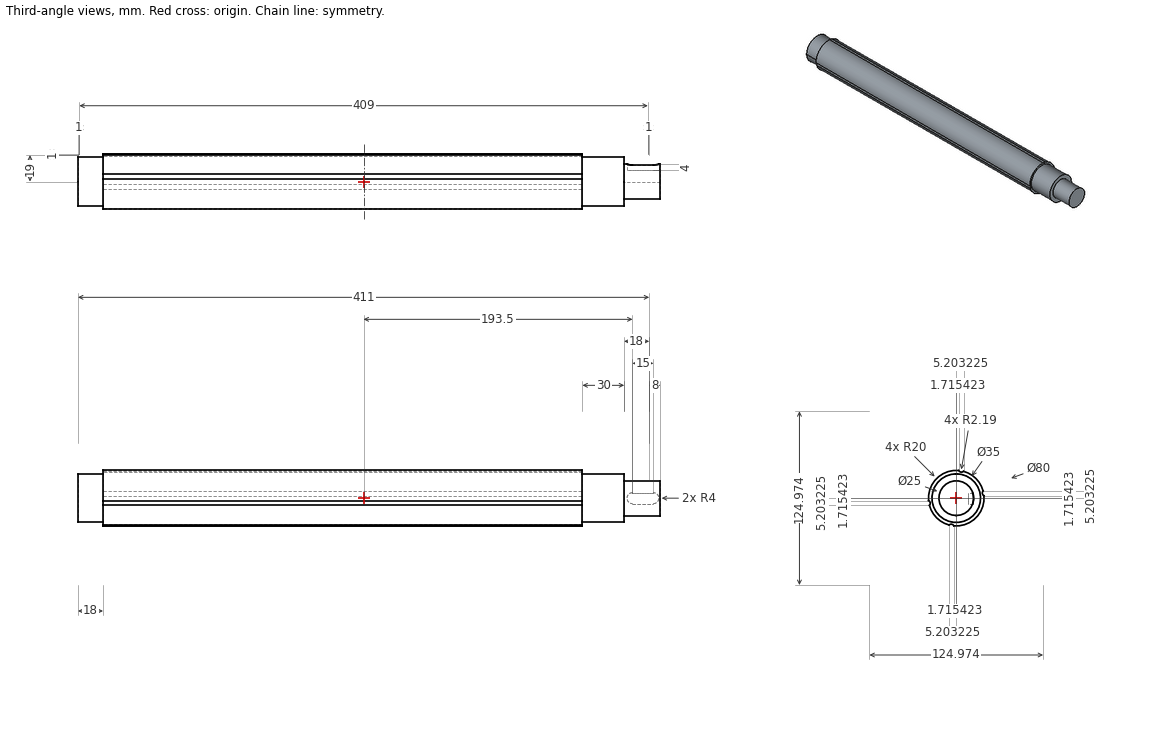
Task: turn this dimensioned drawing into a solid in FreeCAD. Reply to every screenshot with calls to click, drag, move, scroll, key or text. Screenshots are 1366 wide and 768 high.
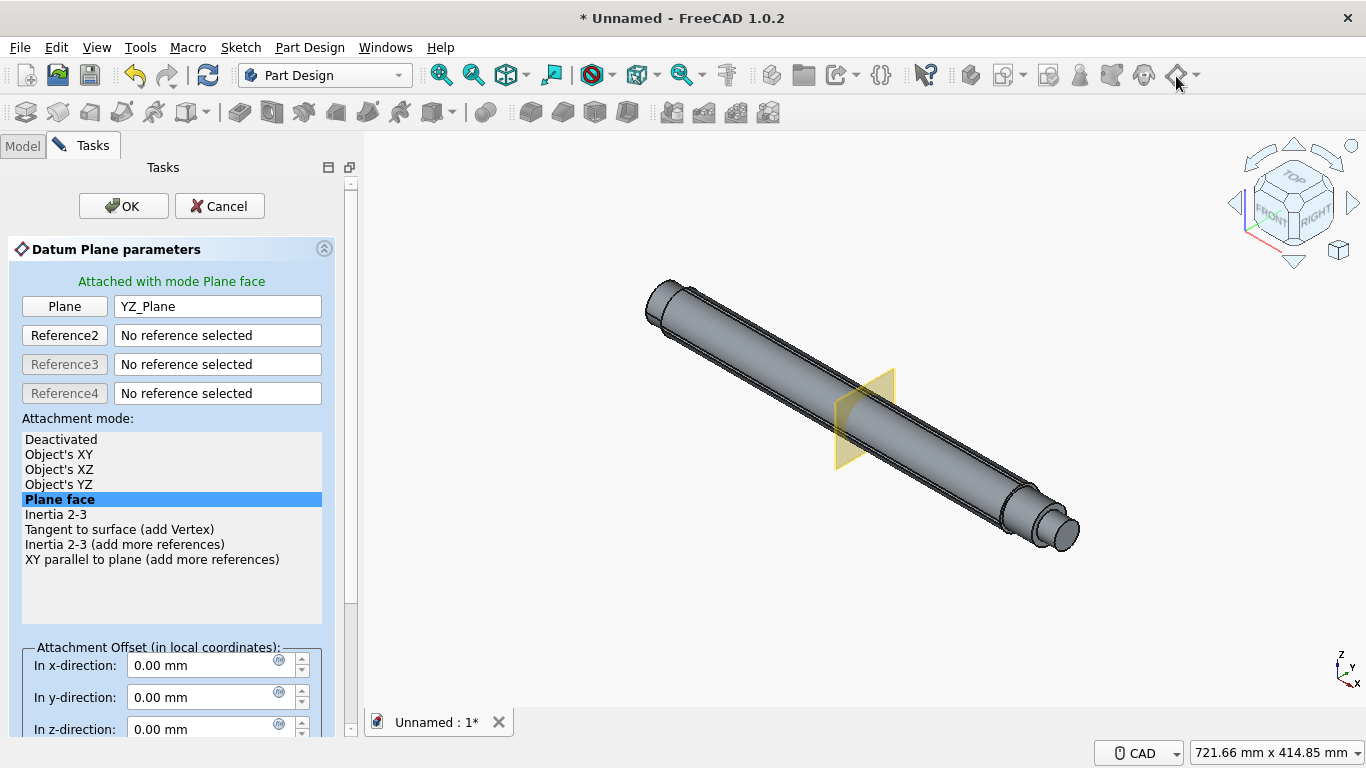
scroll(351, 456, down, 2)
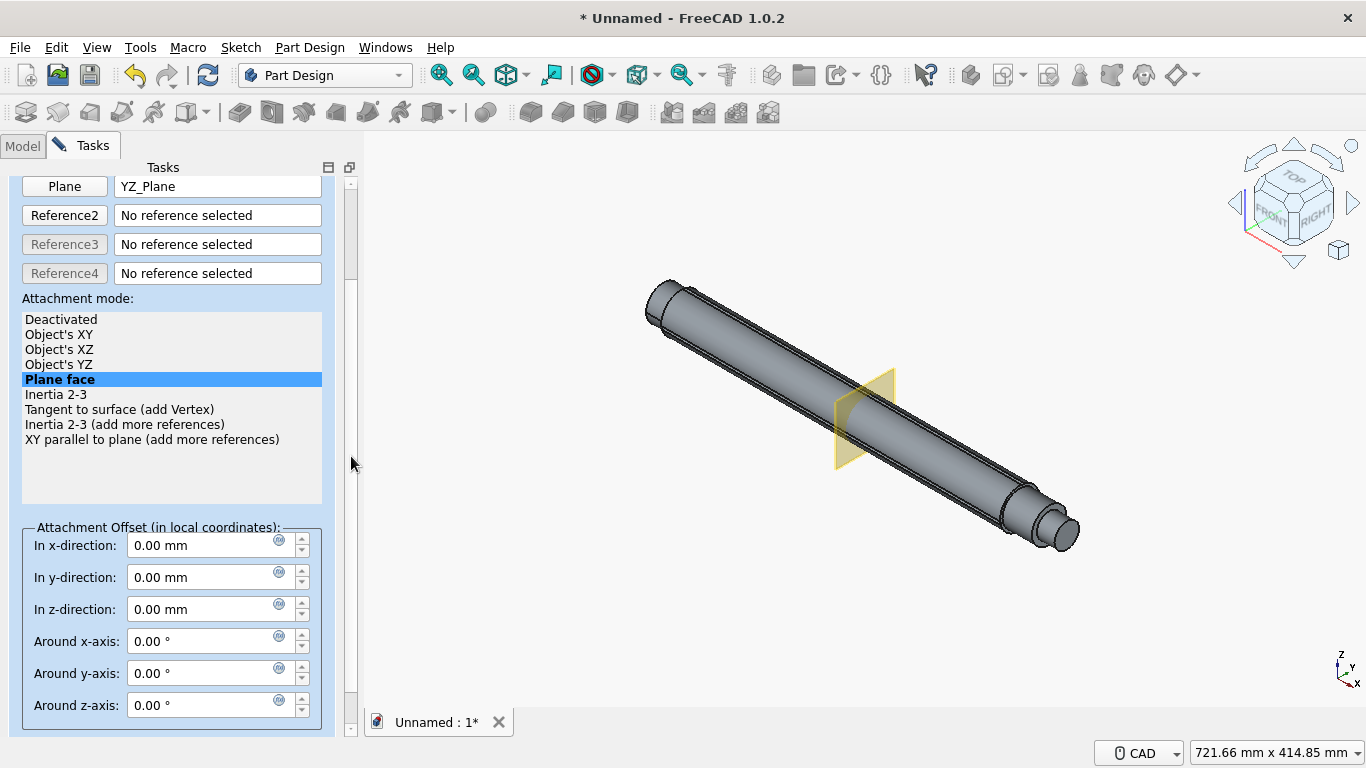
triple_click(210, 609)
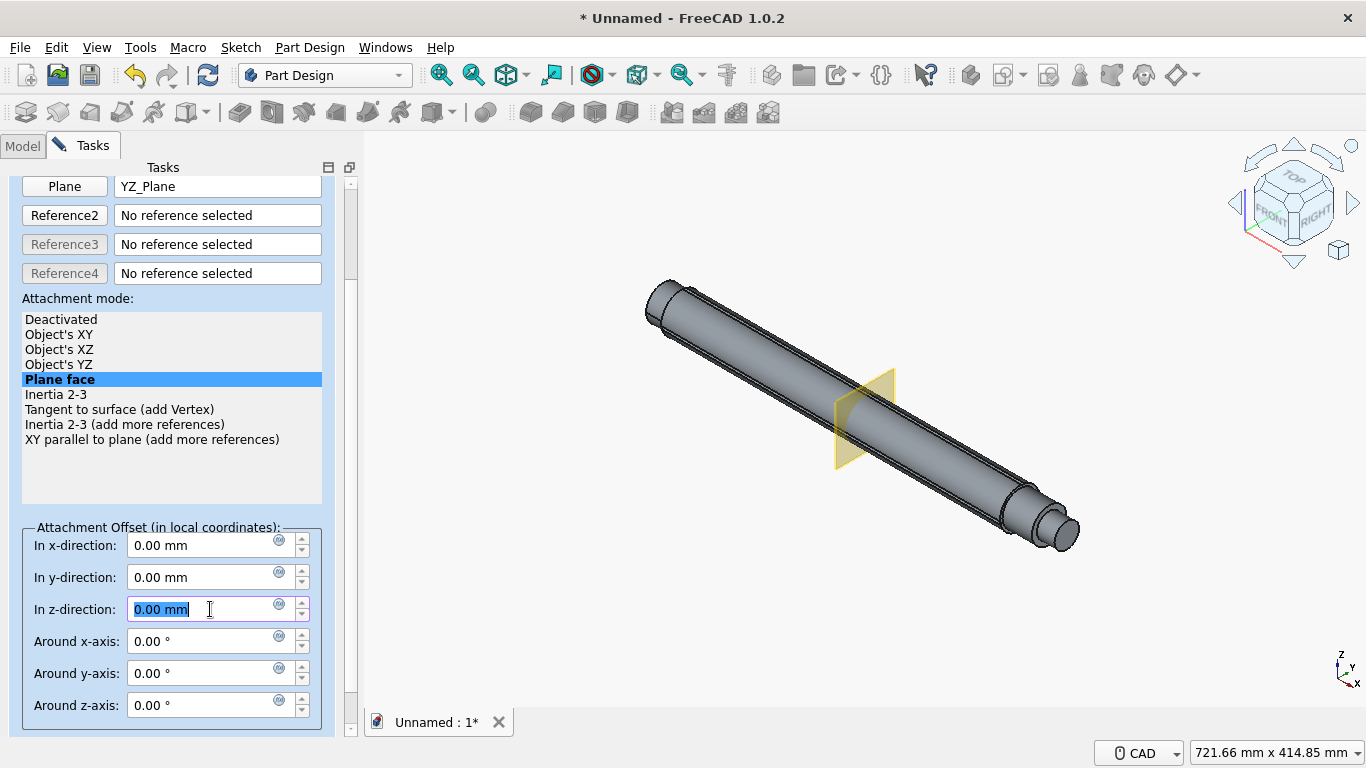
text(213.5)
key(Tab)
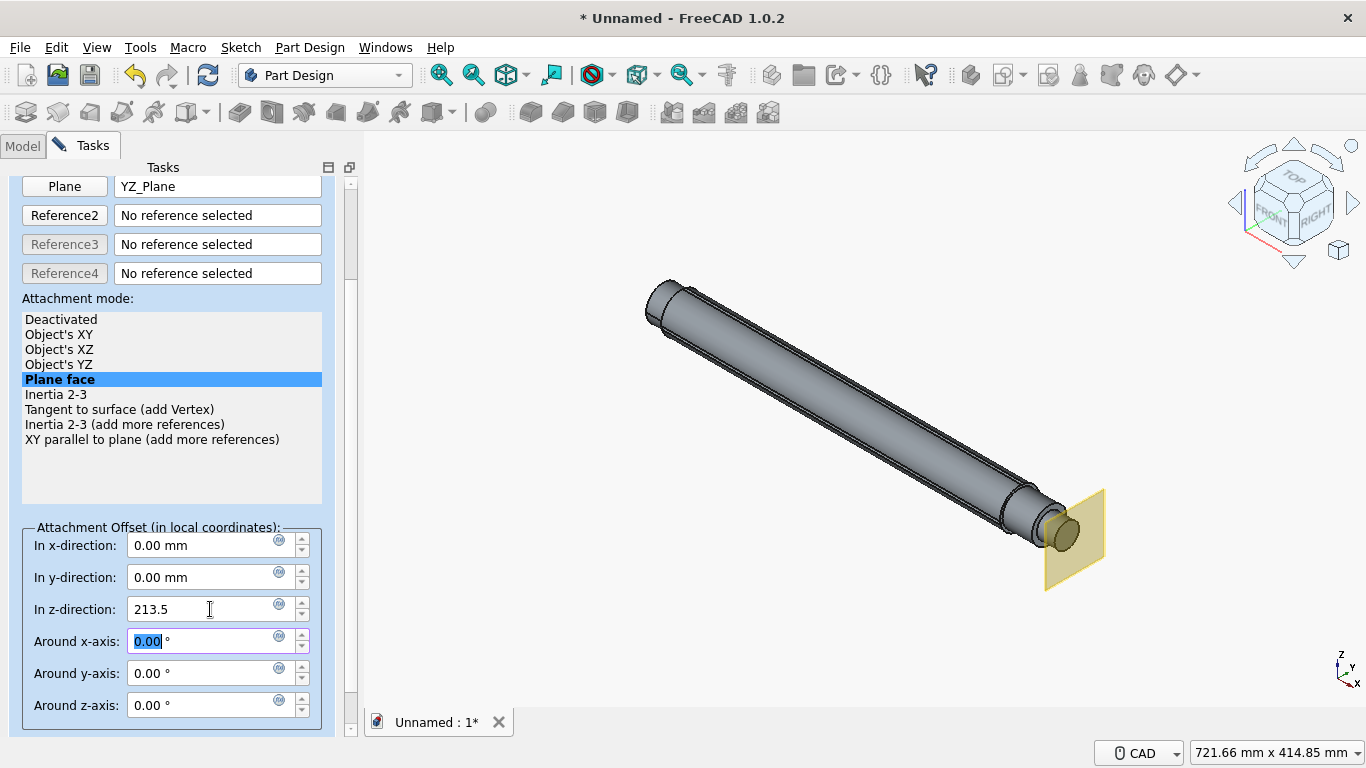
scroll(351, 456, up, 3)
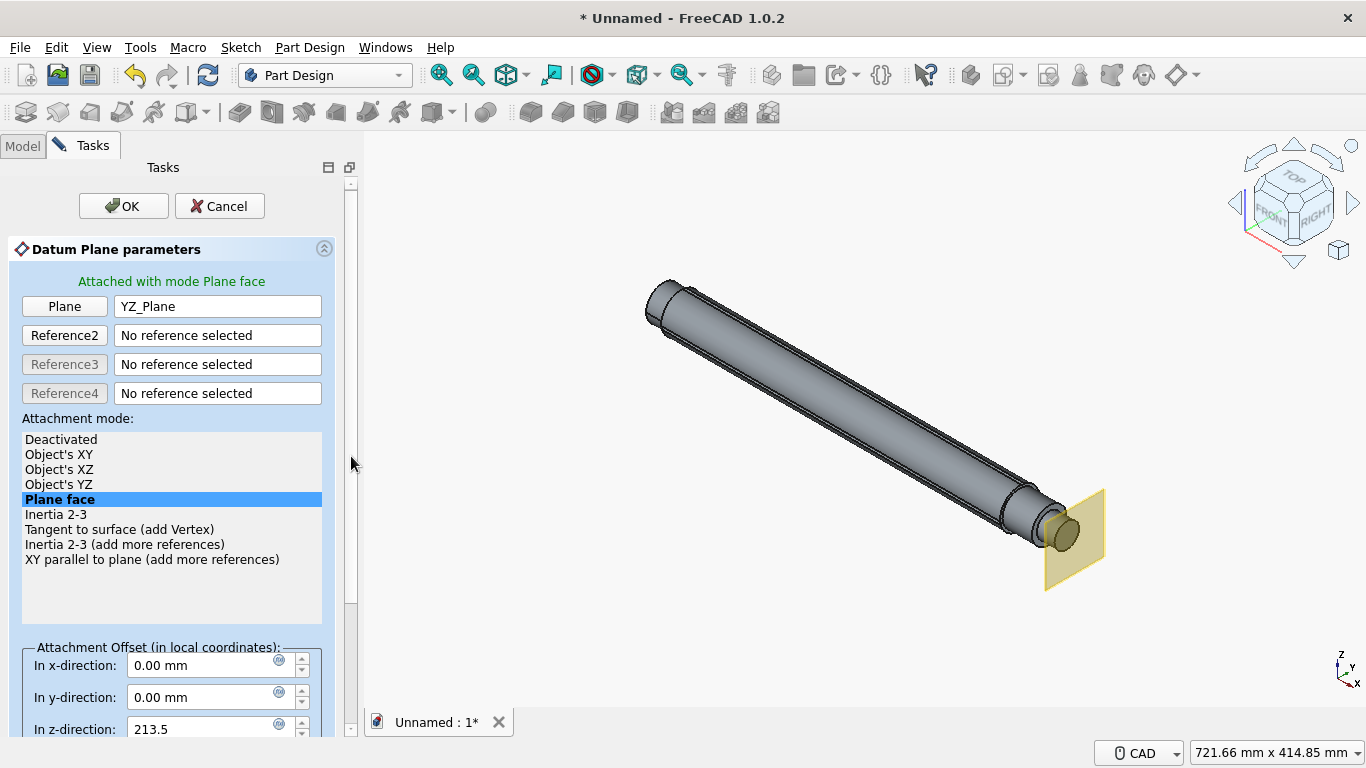
click(124, 206)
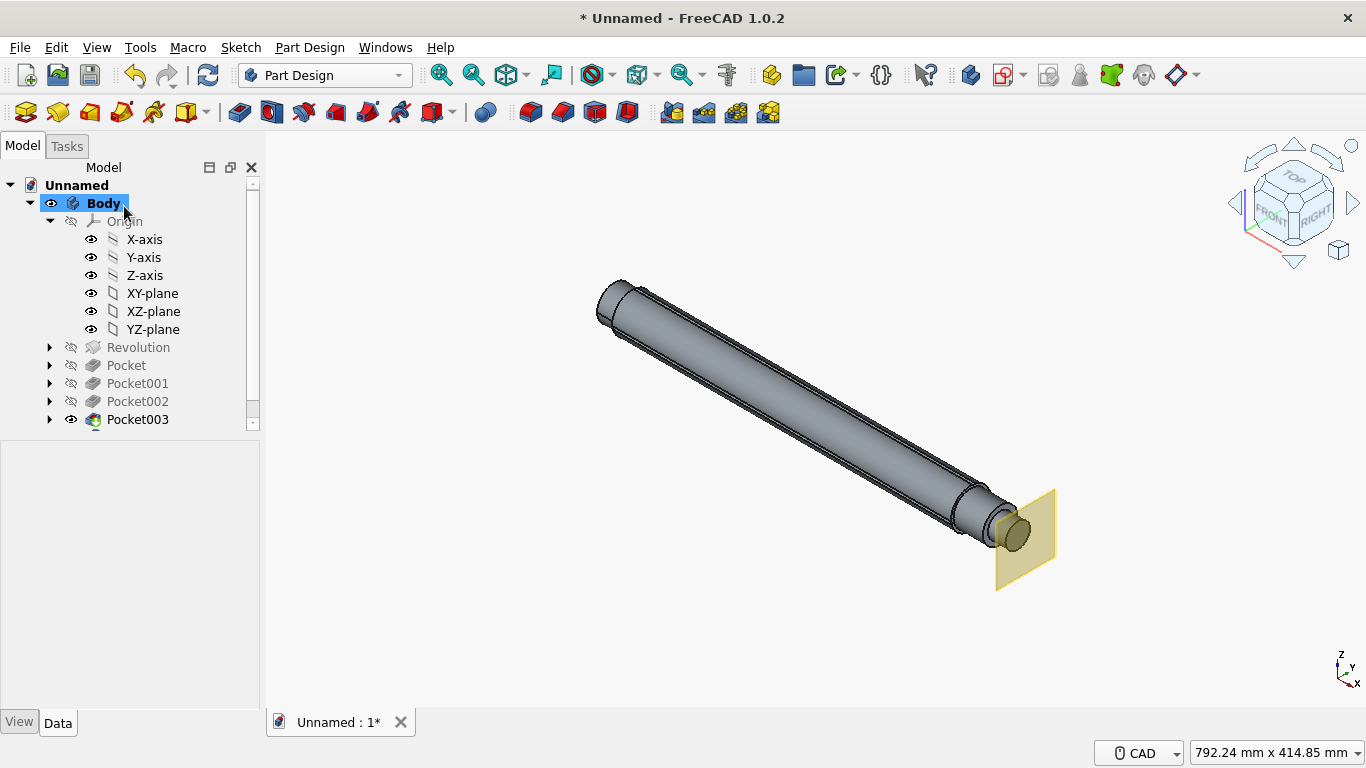
scroll(100, 307, down, 3)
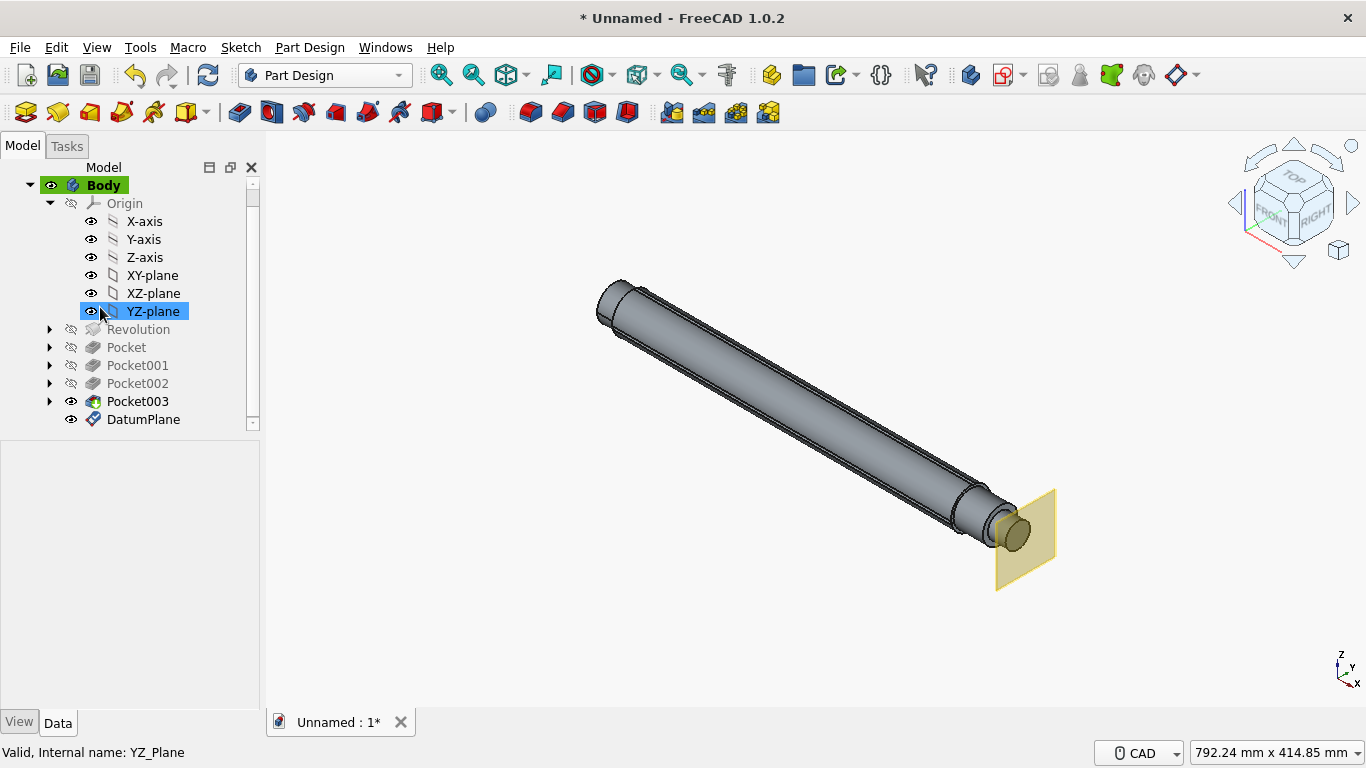
click(116, 419)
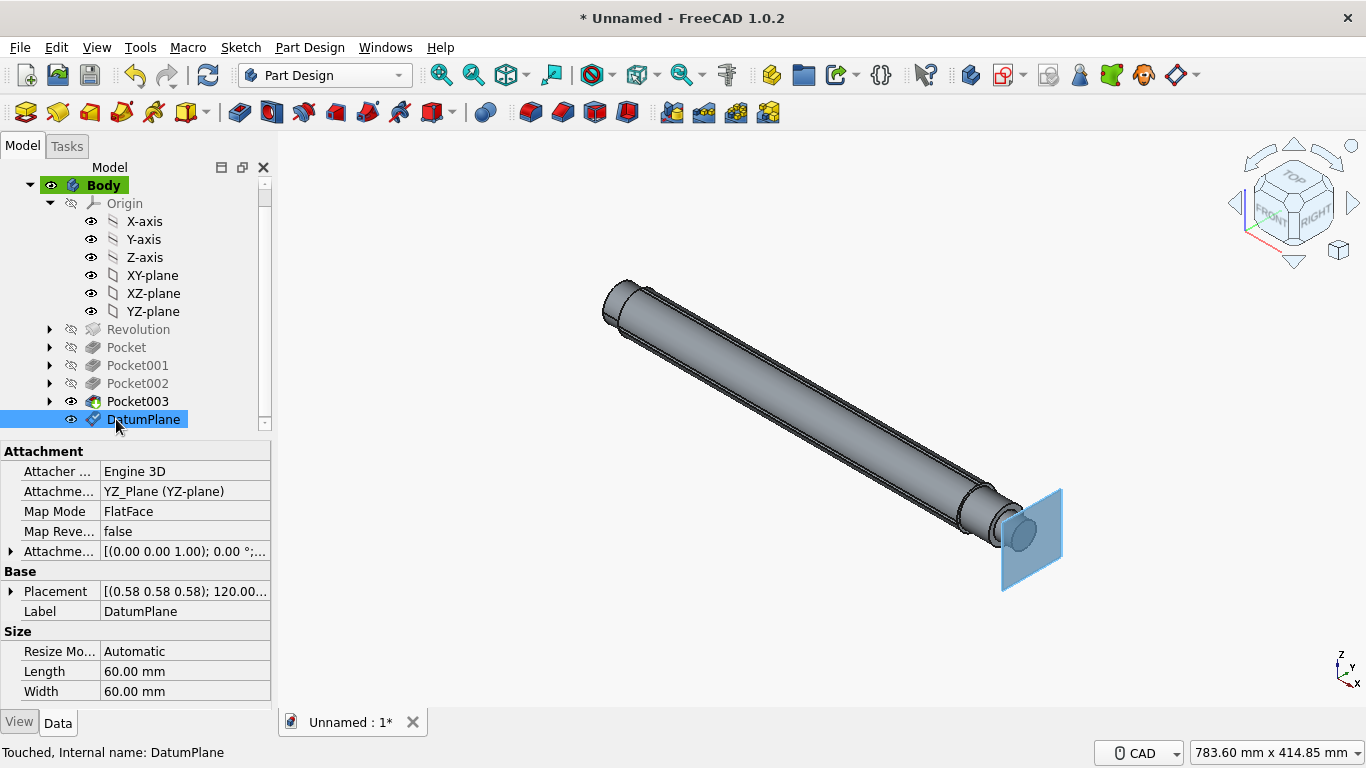
click(1004, 76)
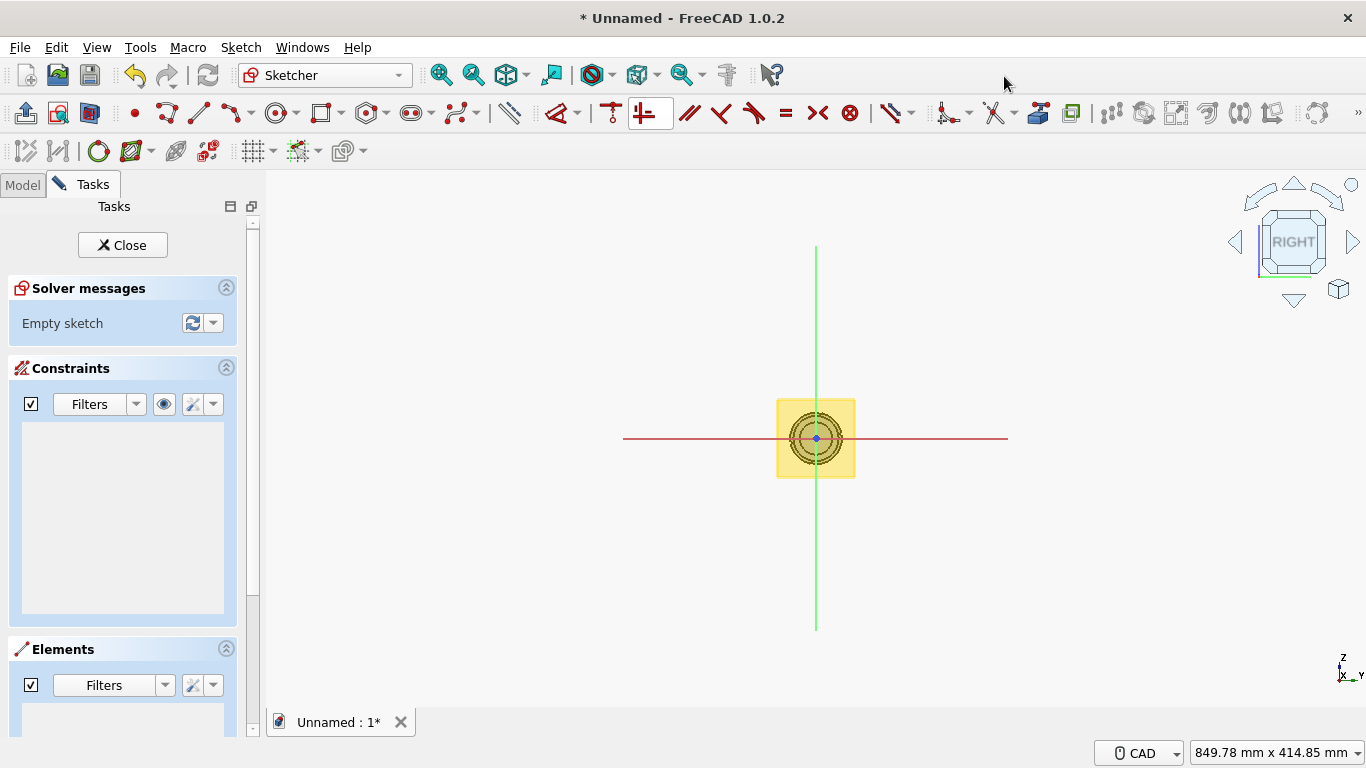
scroll(823, 438, up, 12)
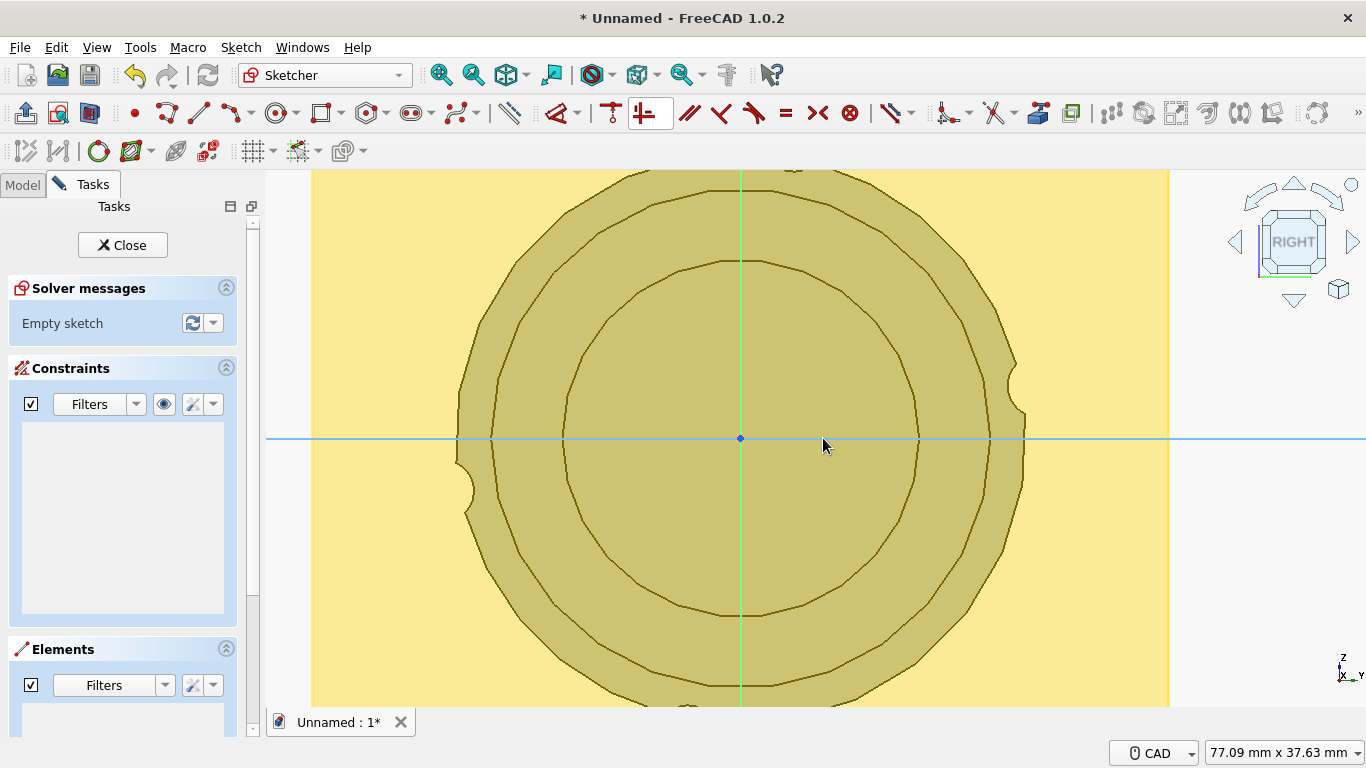
key(g)
key(c)